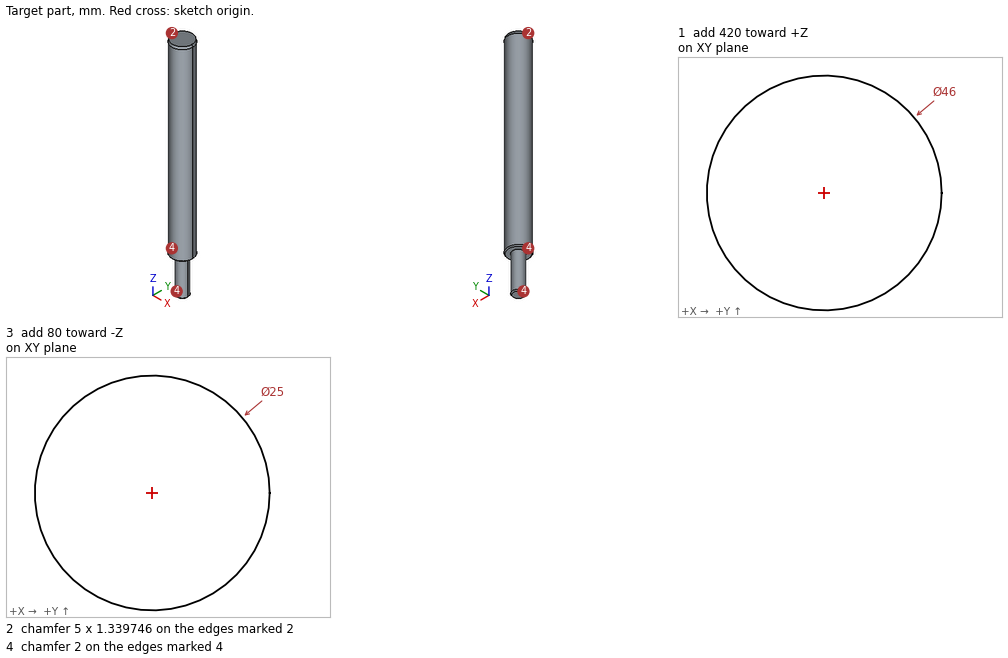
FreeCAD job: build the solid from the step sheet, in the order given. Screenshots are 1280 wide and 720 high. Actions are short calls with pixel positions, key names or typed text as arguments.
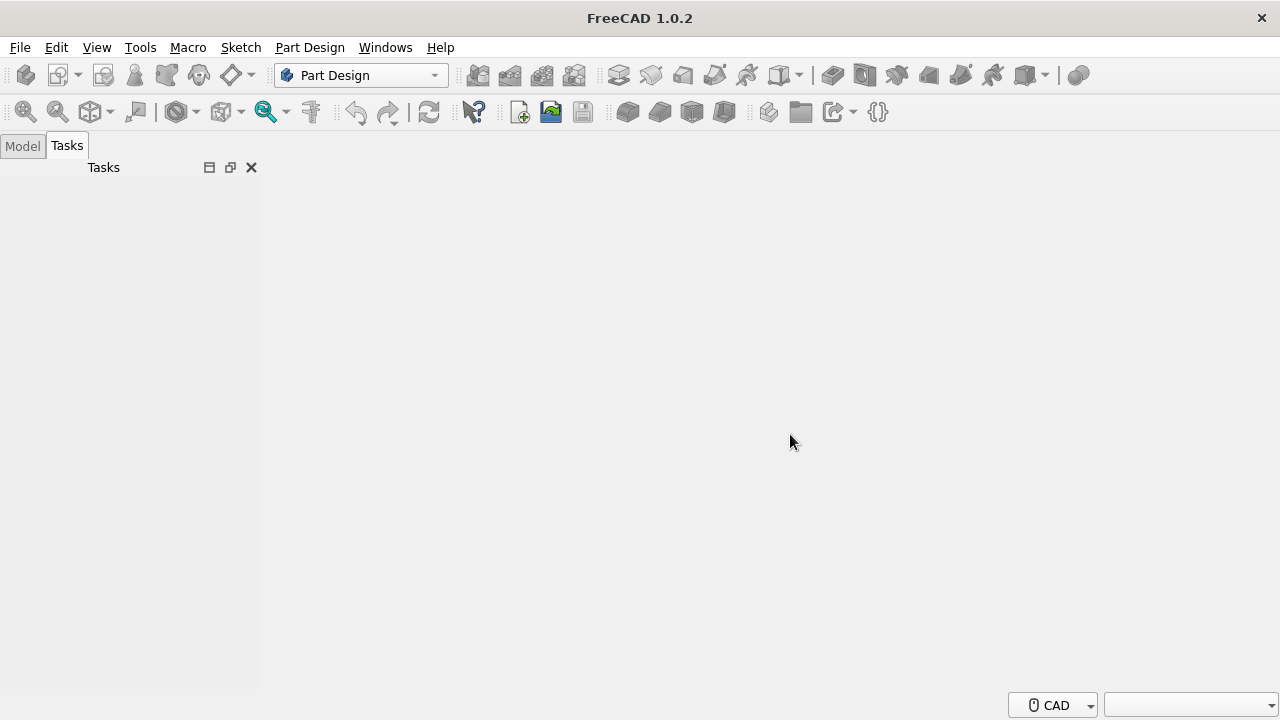
click(520, 112)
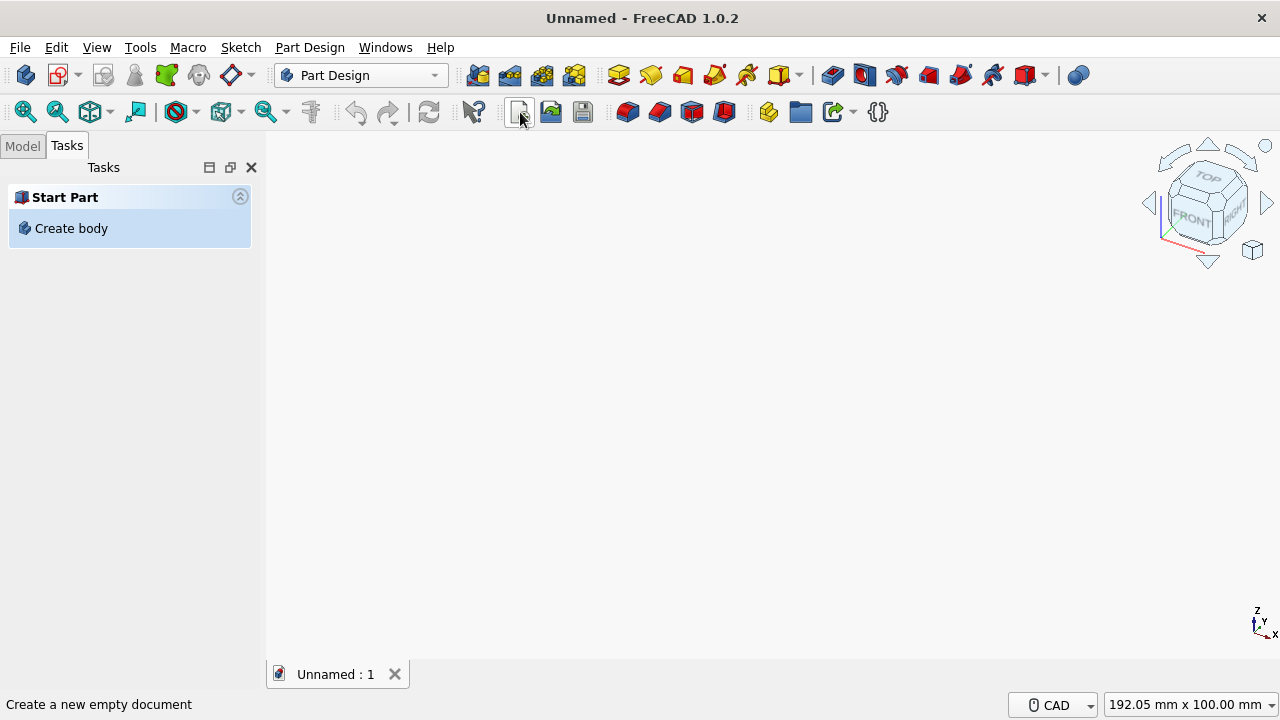
click(58, 76)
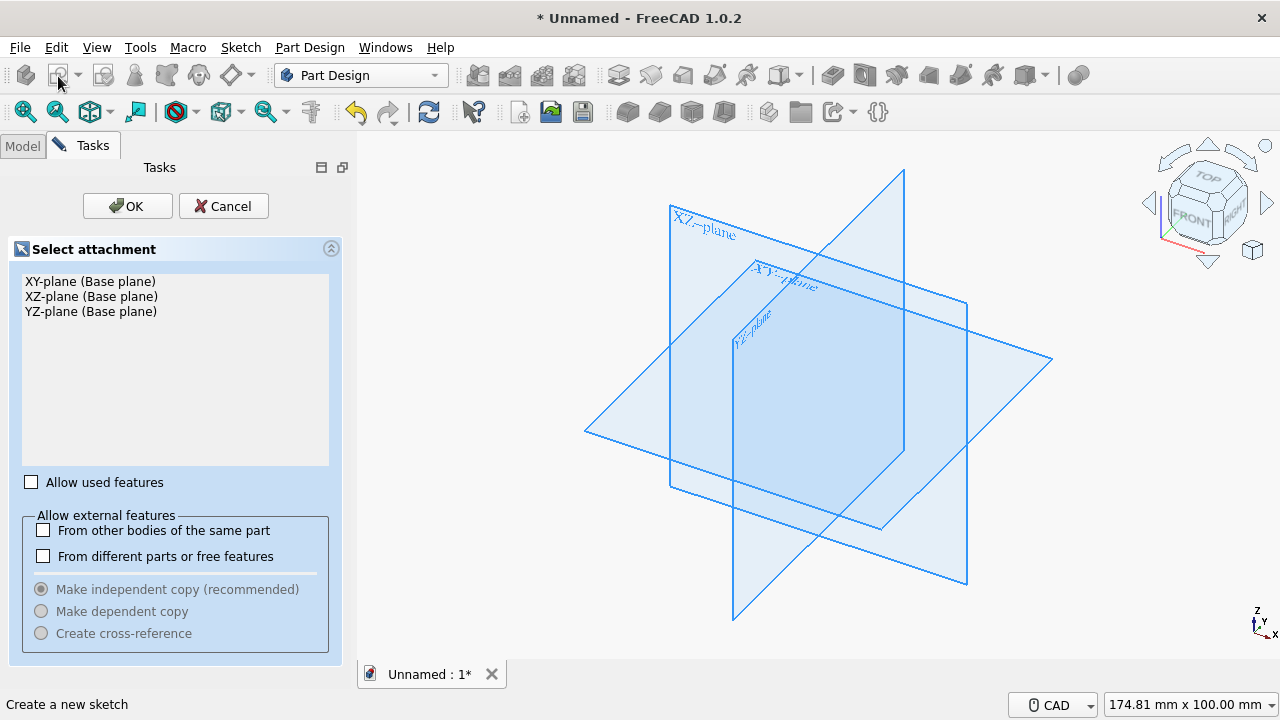
click(82, 282)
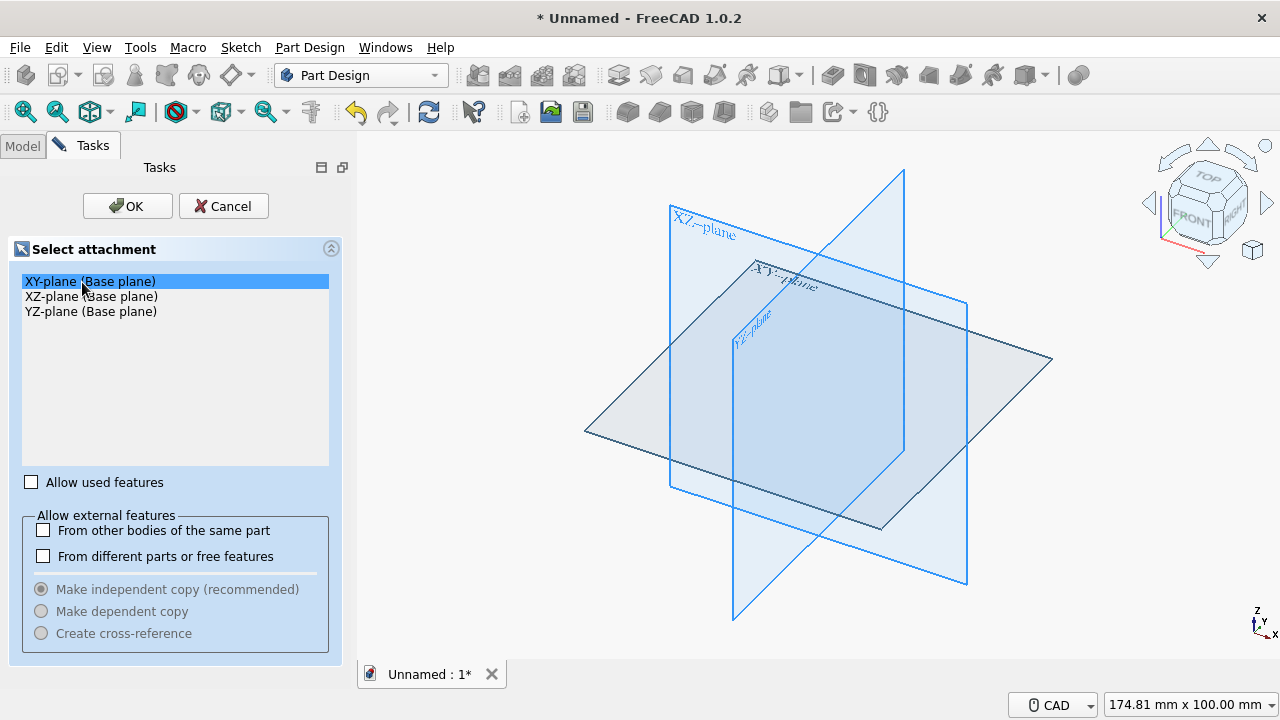
click(128, 206)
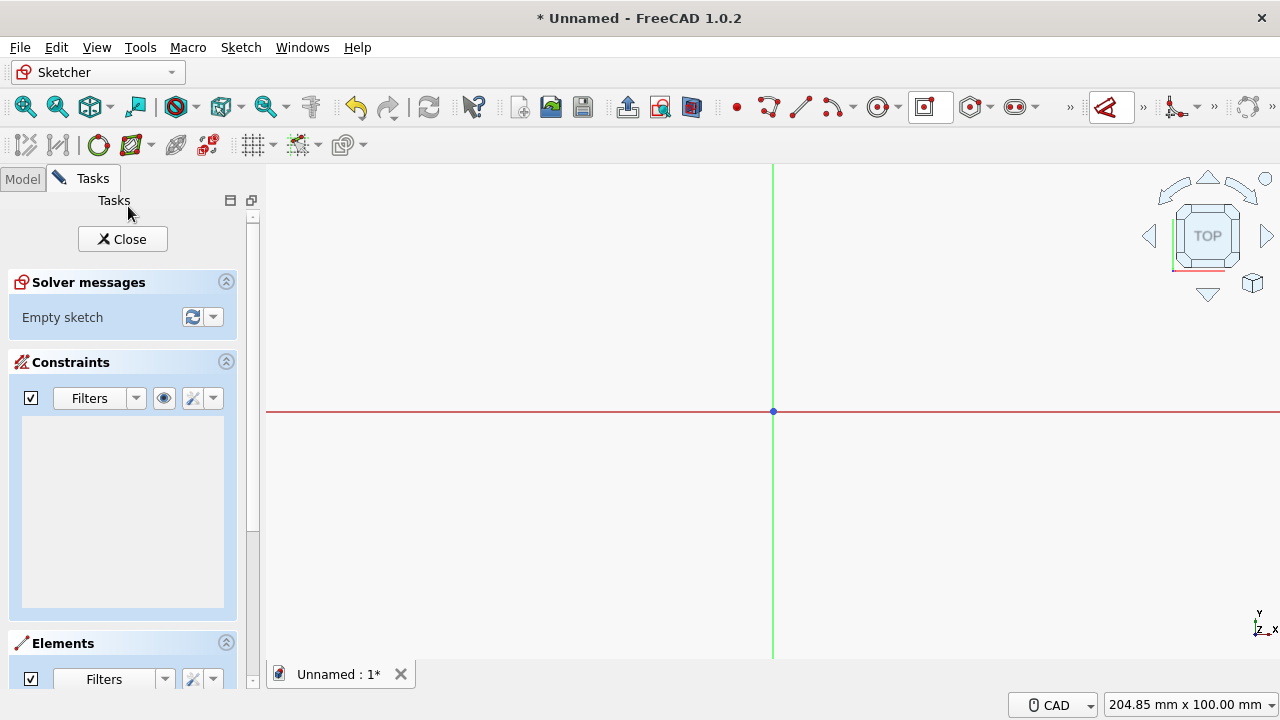
scroll(912, 411, up, 2)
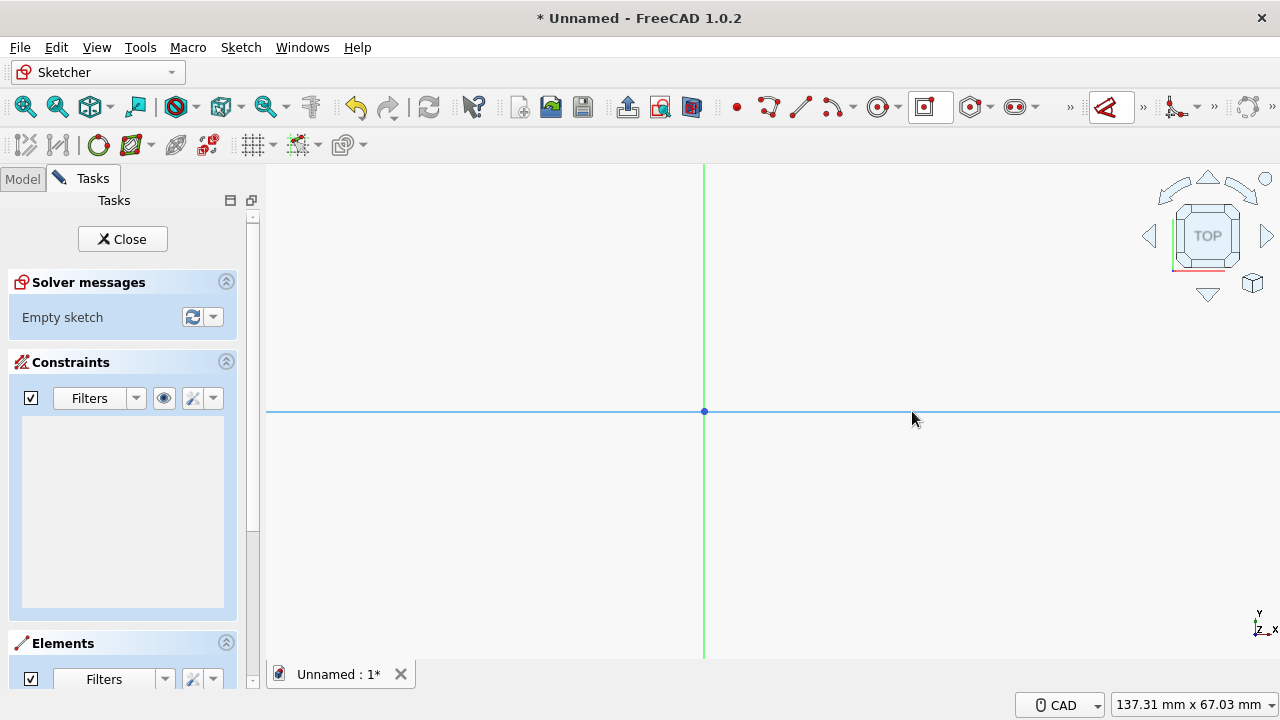
click(878, 108)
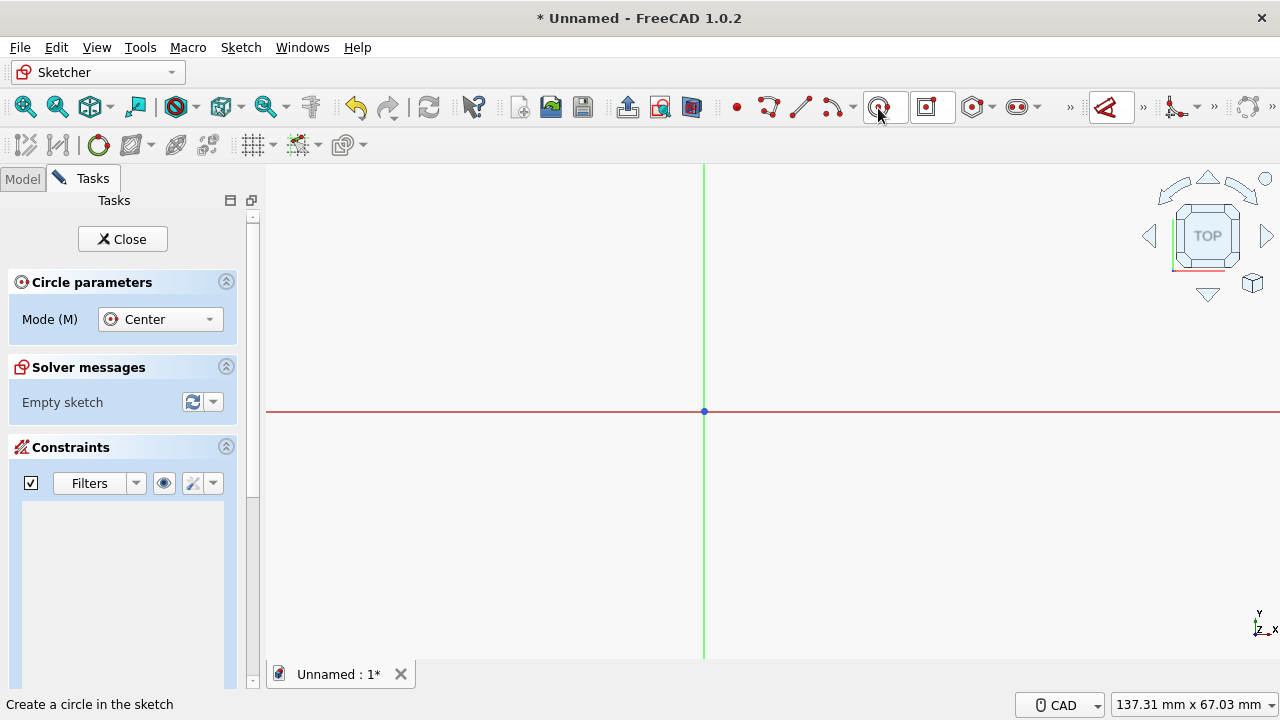
click(704, 412)
move(824, 291)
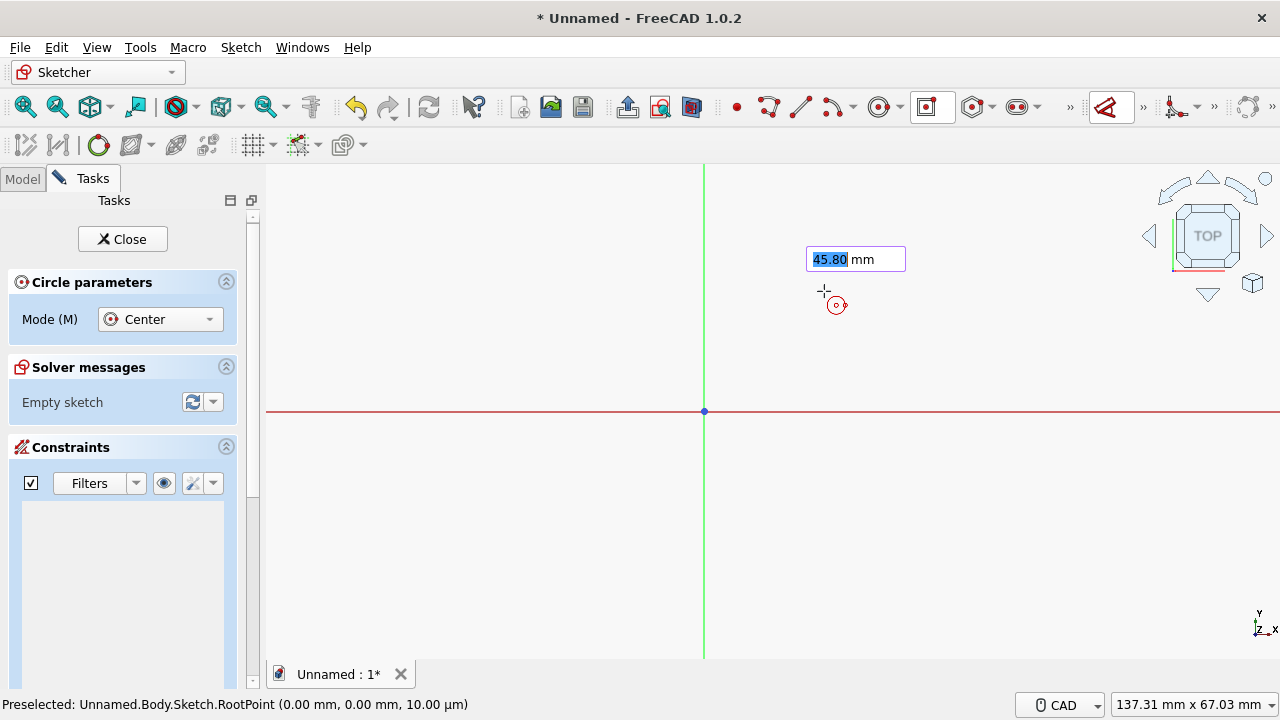
text(46)
key(Return)
key(Escape)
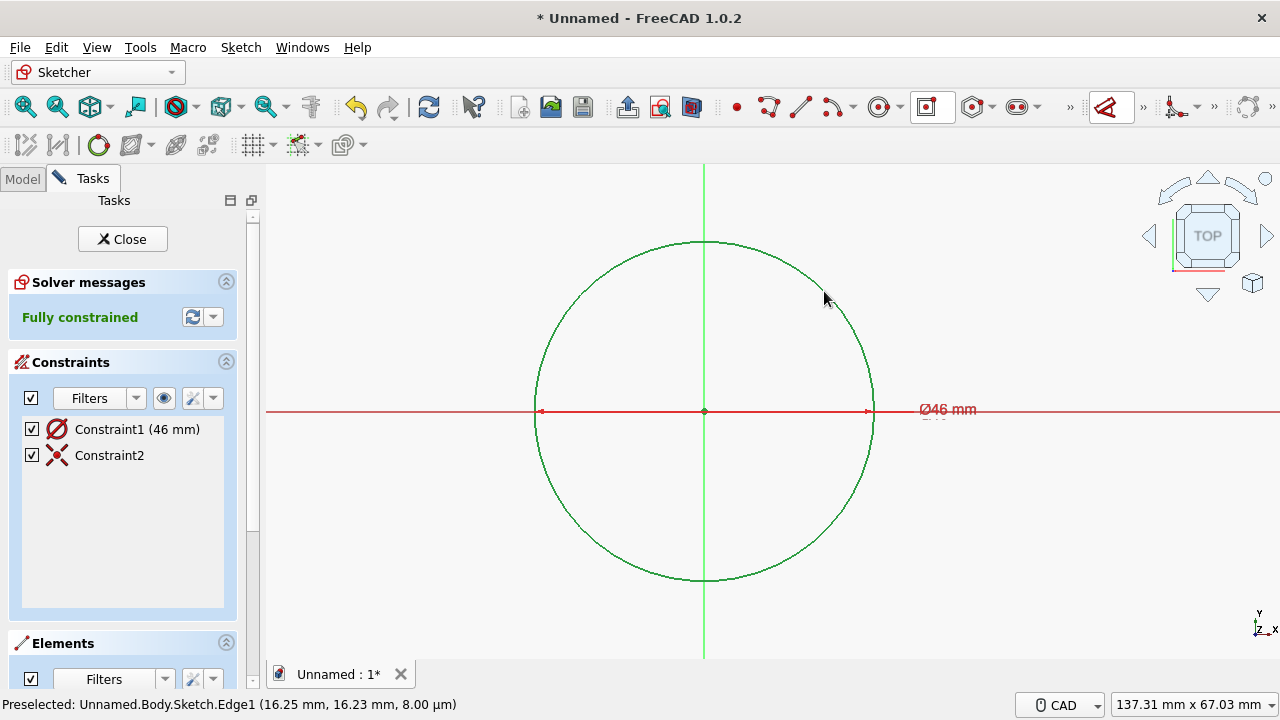
click(123, 239)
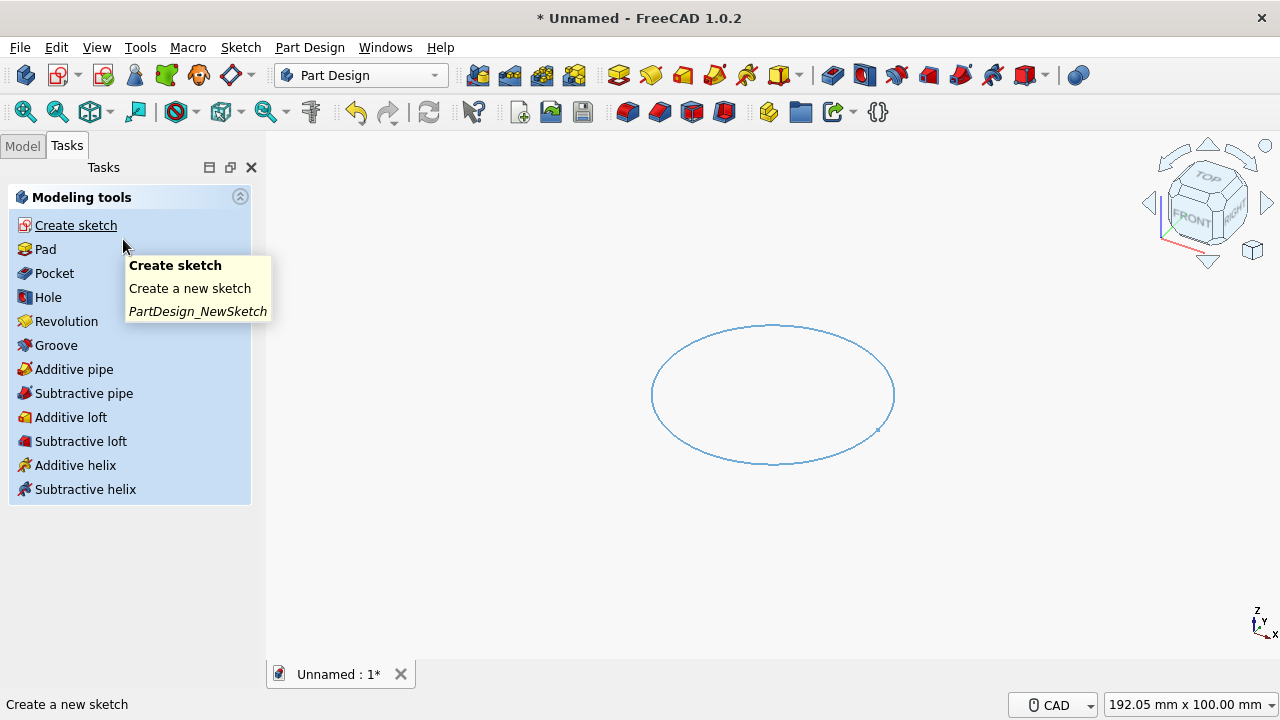
click(620, 76)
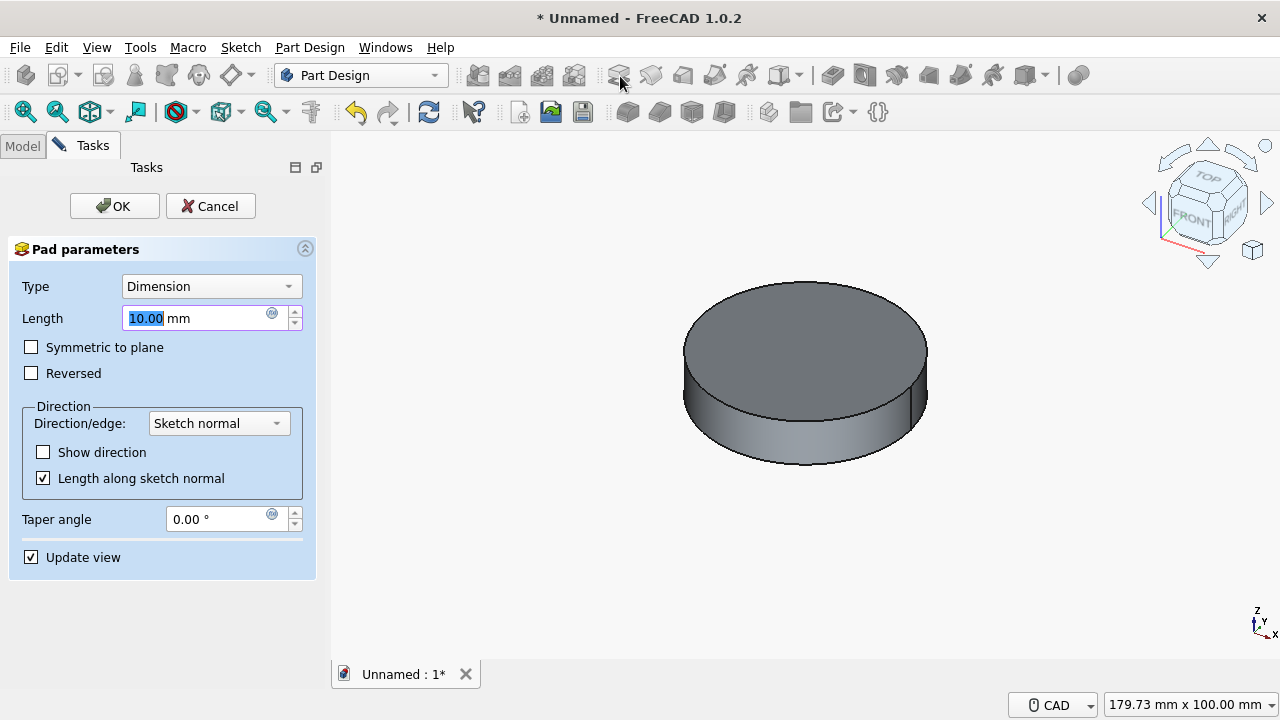
text(420)
key(Tab)